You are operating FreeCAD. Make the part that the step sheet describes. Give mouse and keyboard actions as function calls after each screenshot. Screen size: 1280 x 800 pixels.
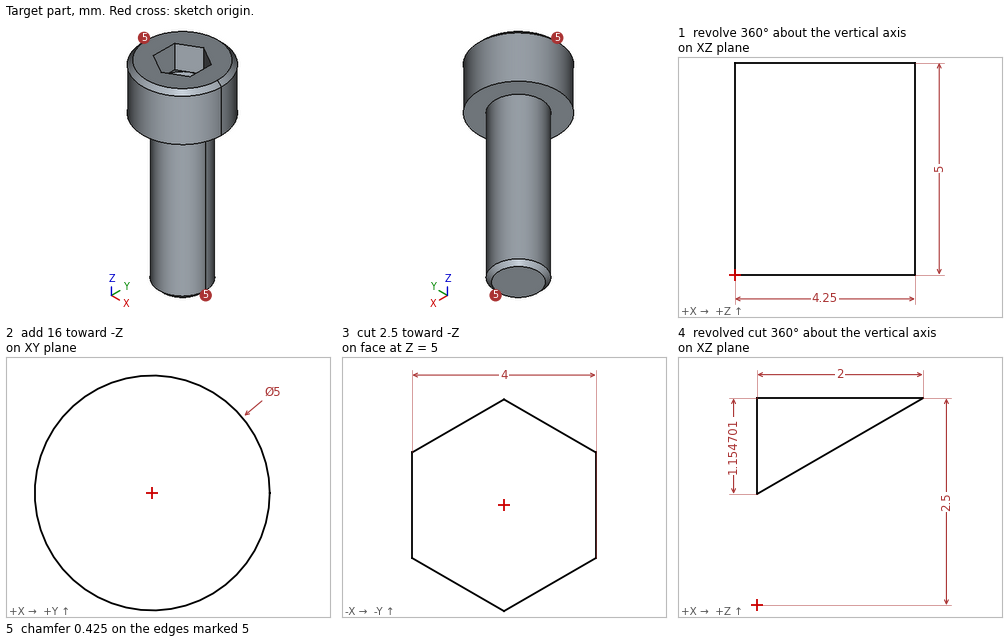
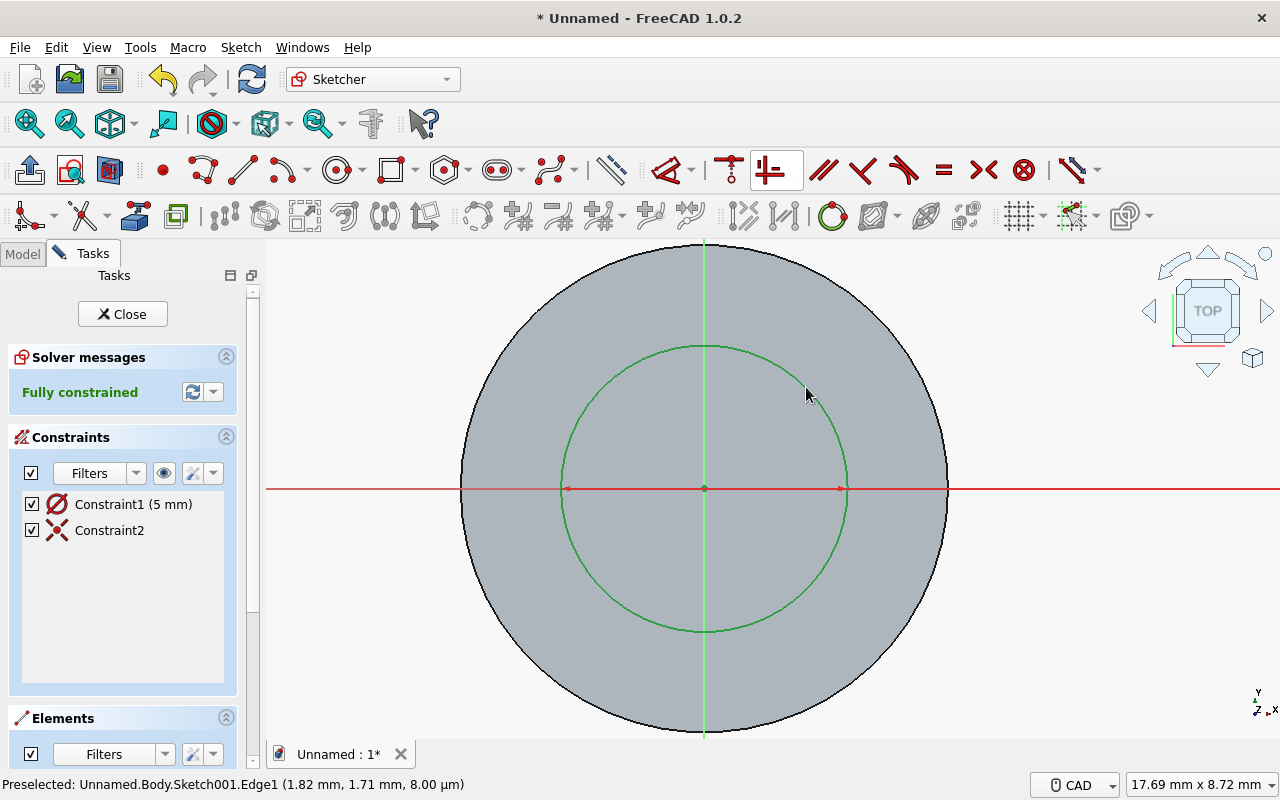
click(123, 314)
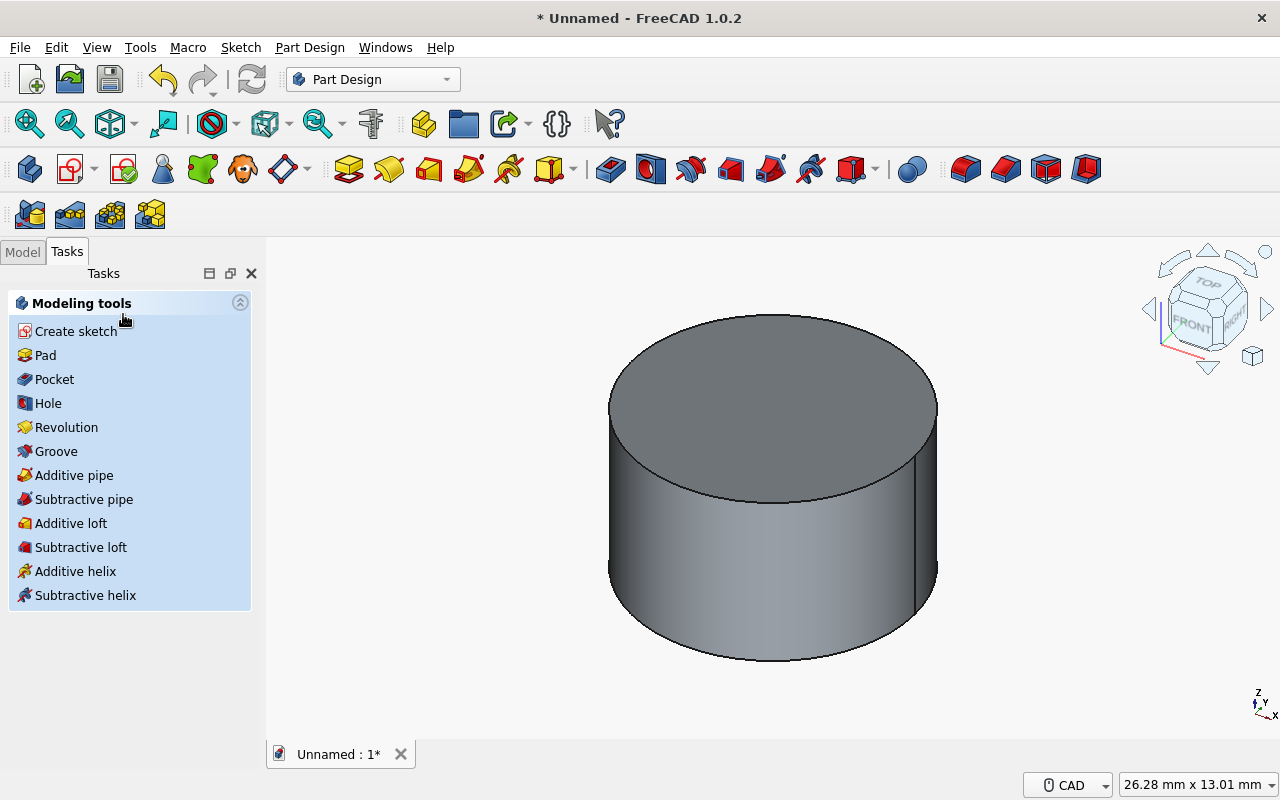
click(350, 170)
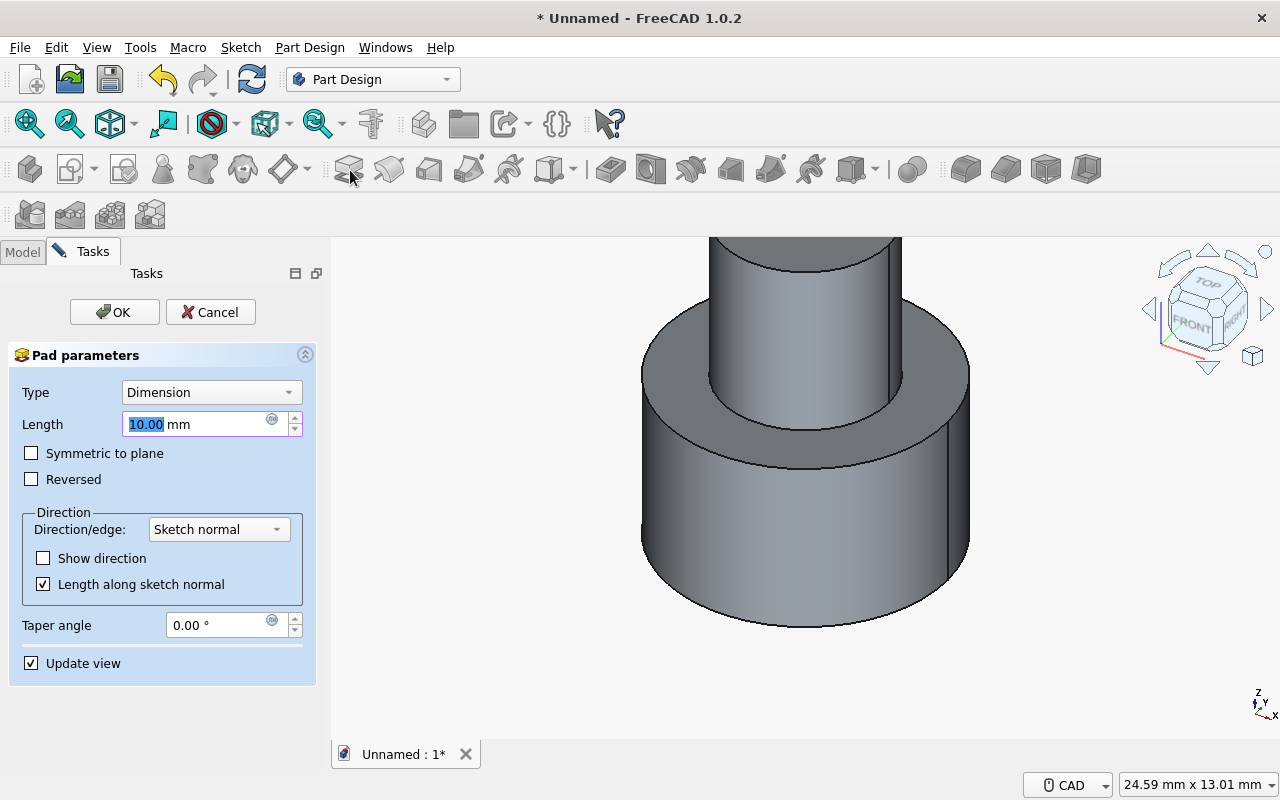
text(16)
key(Tab)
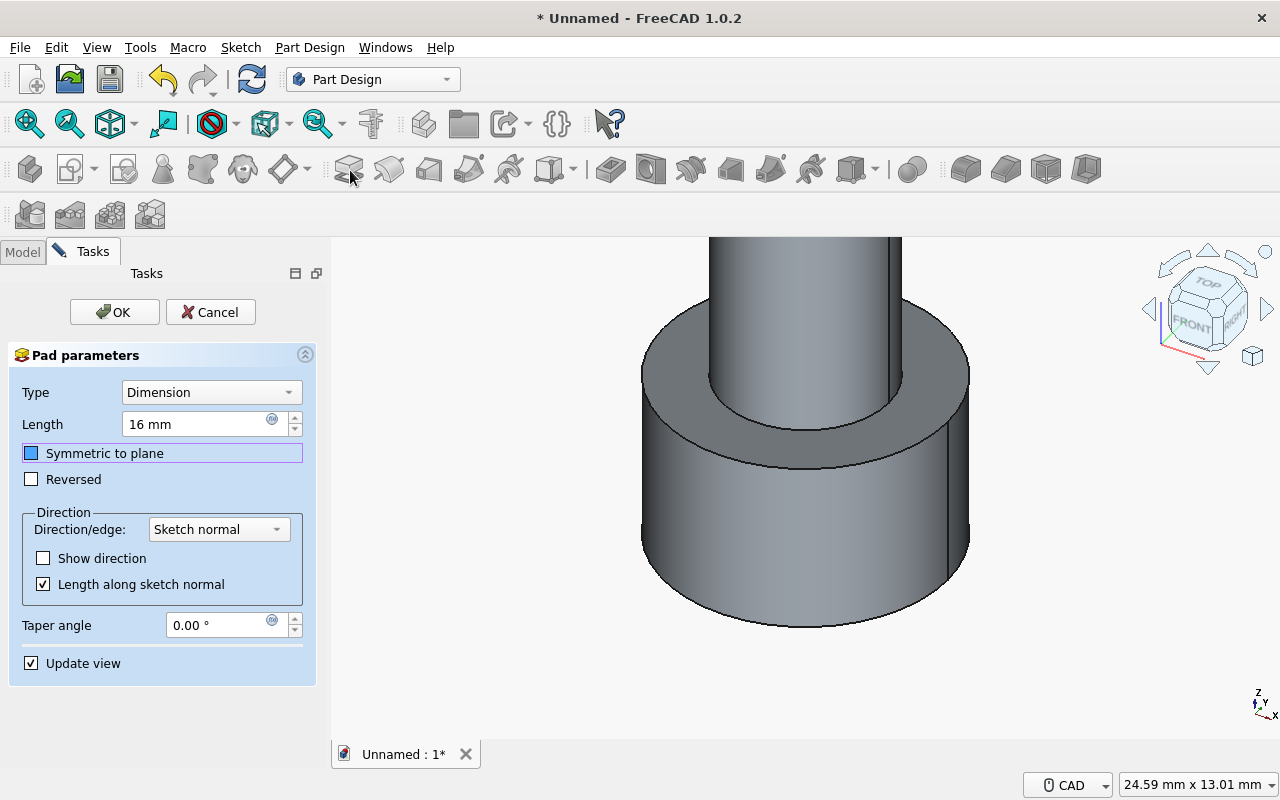
click(30, 479)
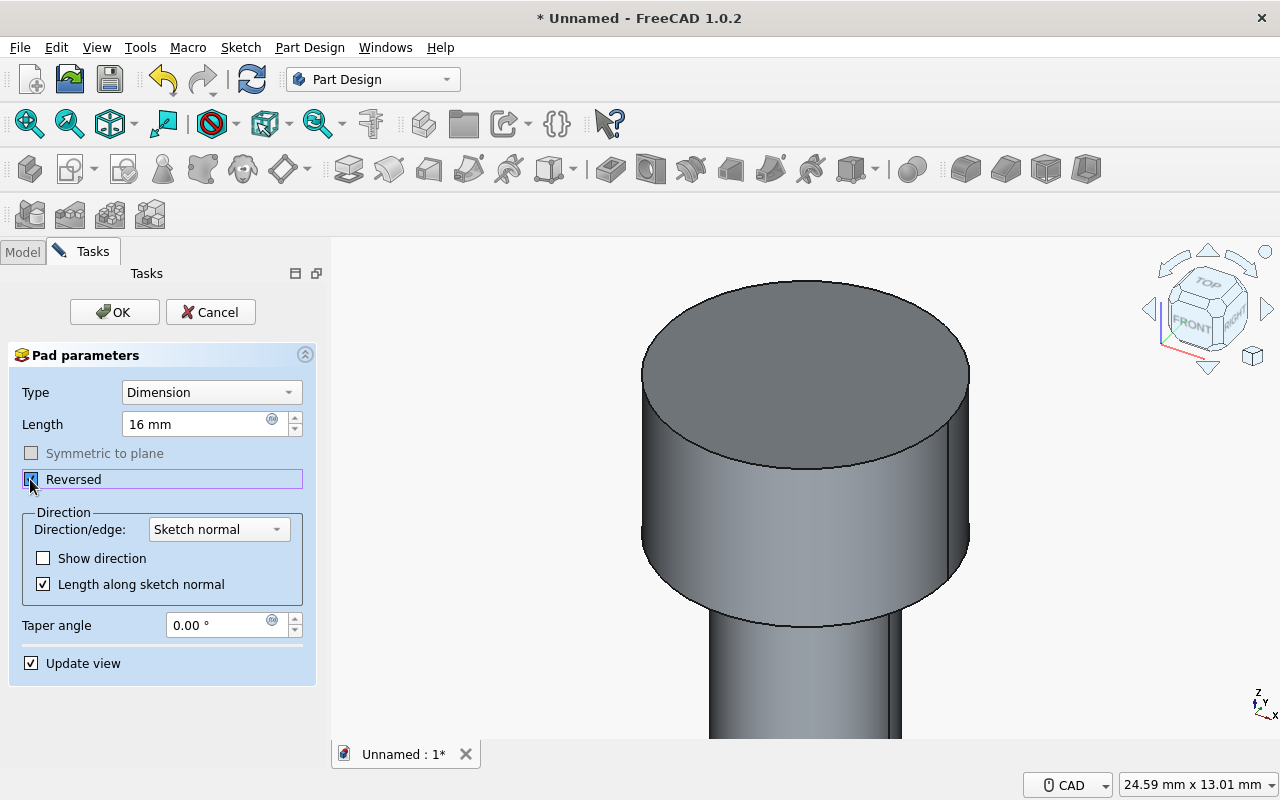
click(115, 312)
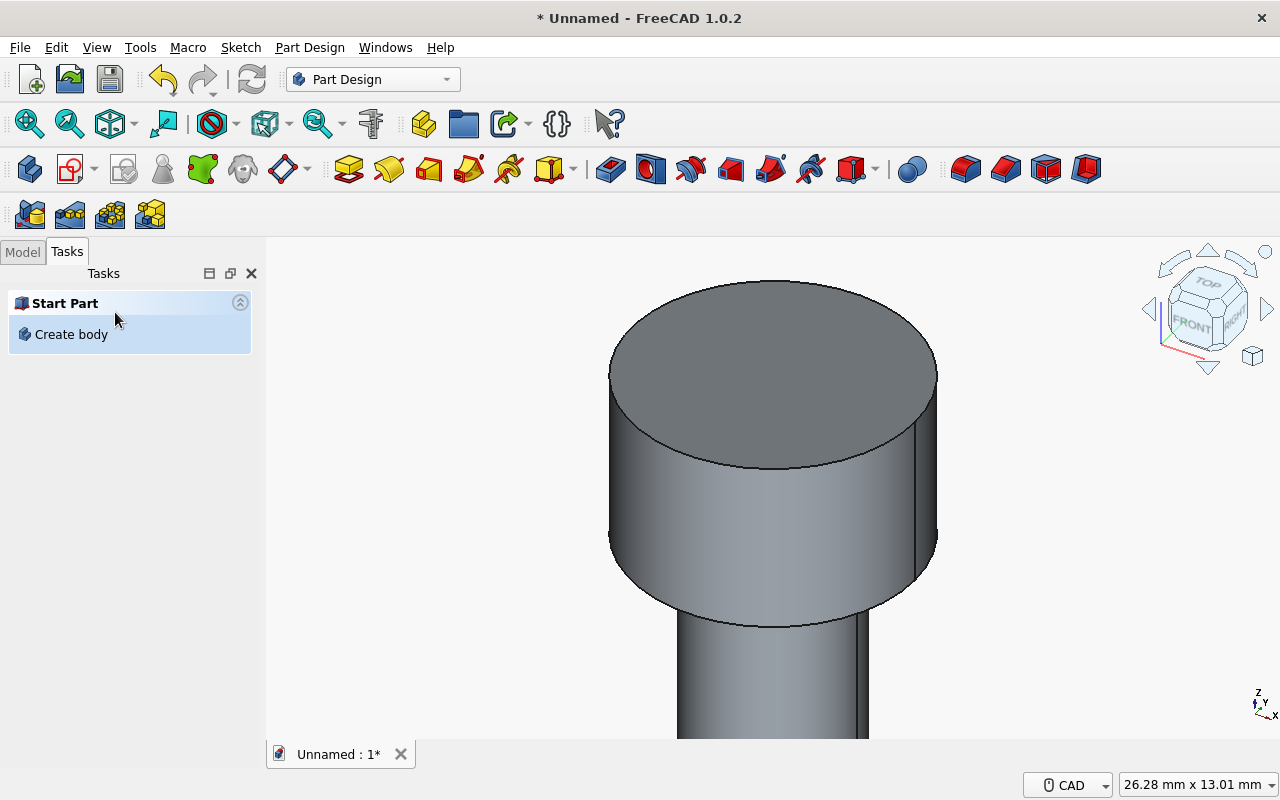
click(30, 124)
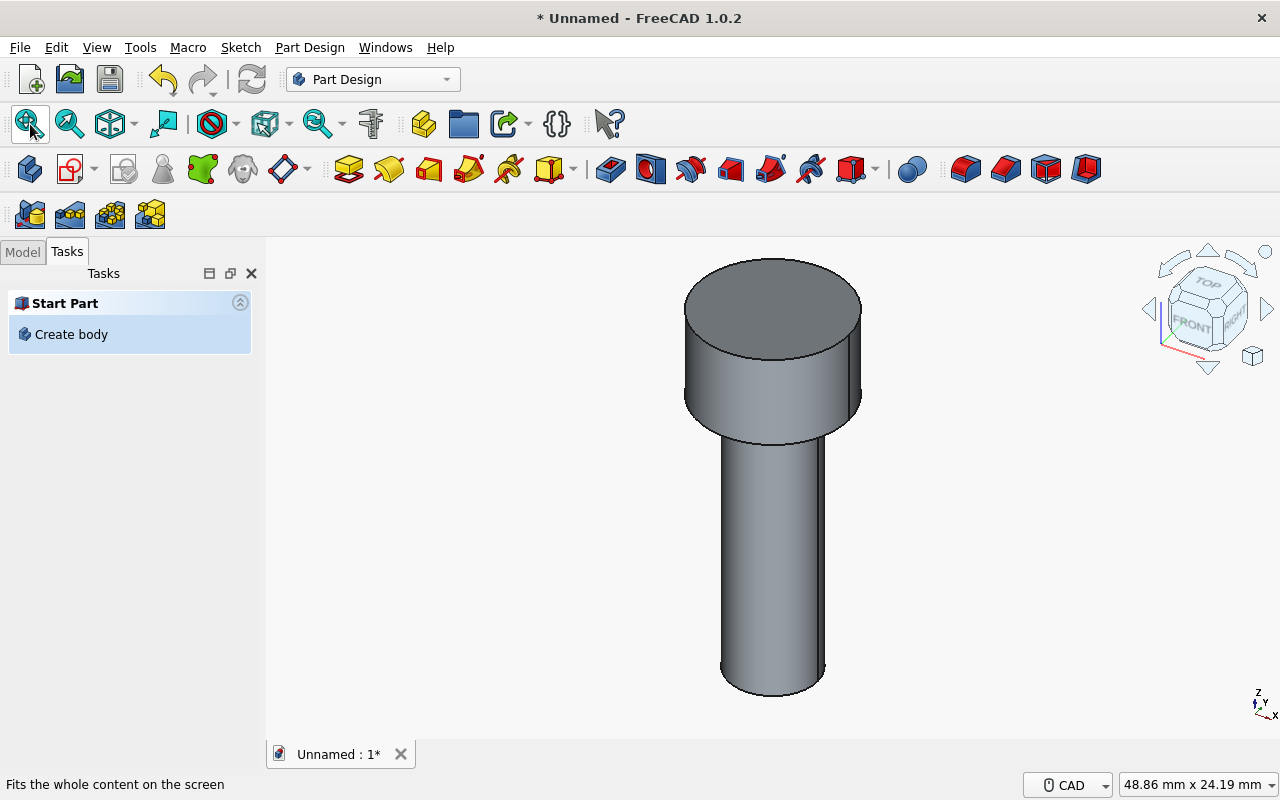
click(773, 308)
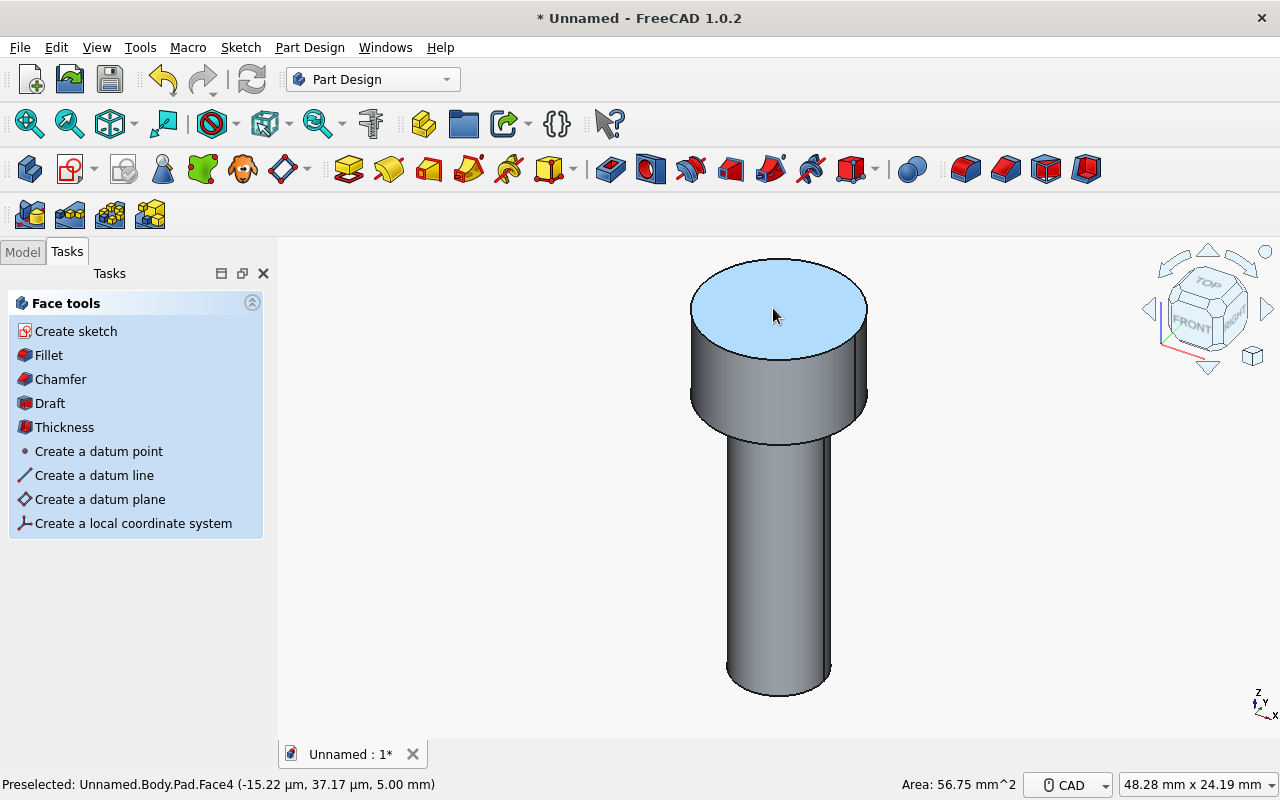
click(70, 170)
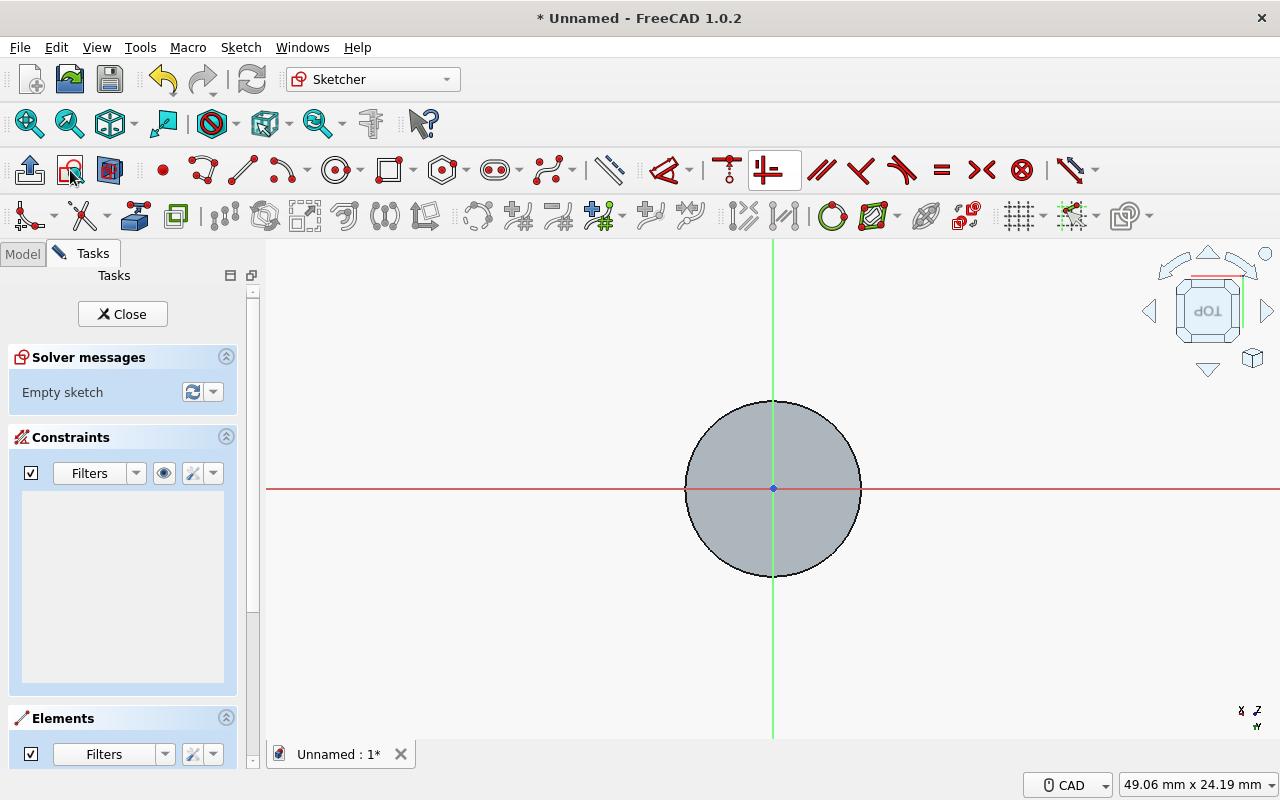
scroll(803, 489, up, 6)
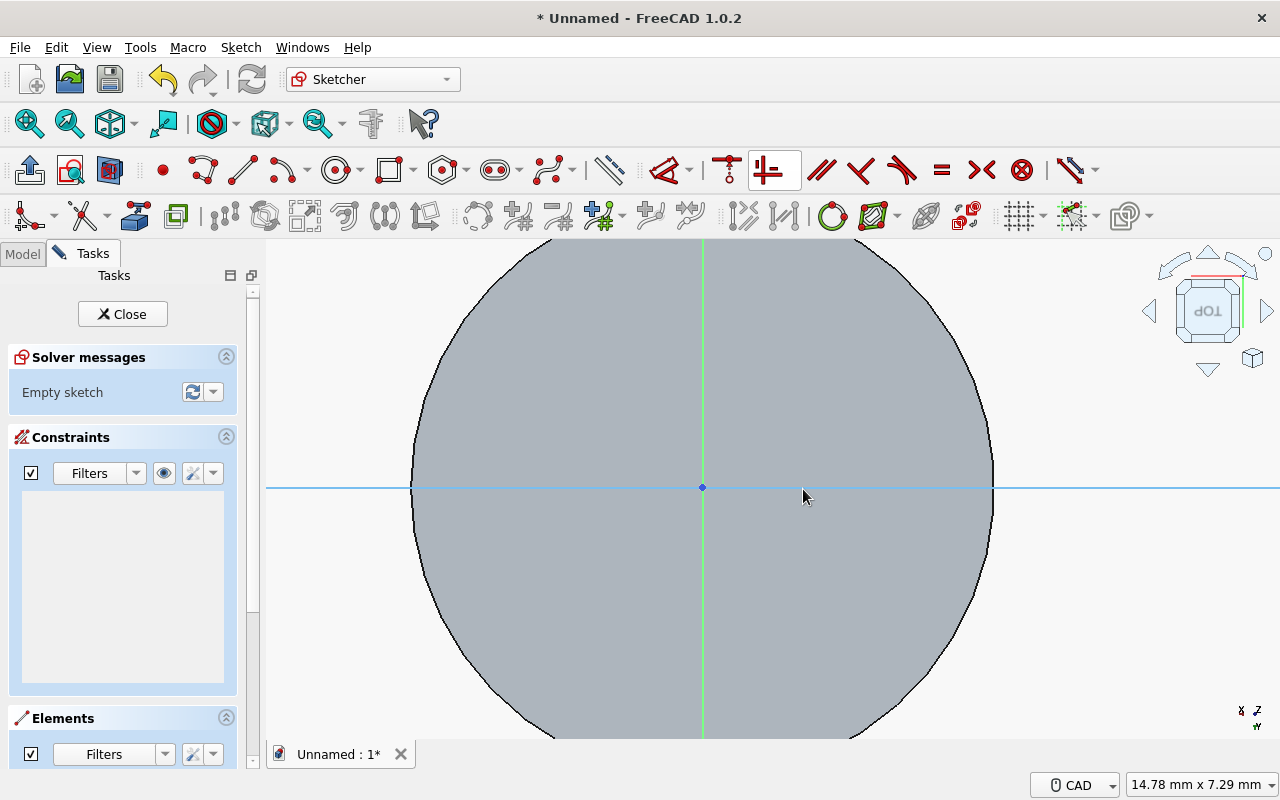
click(442, 170)